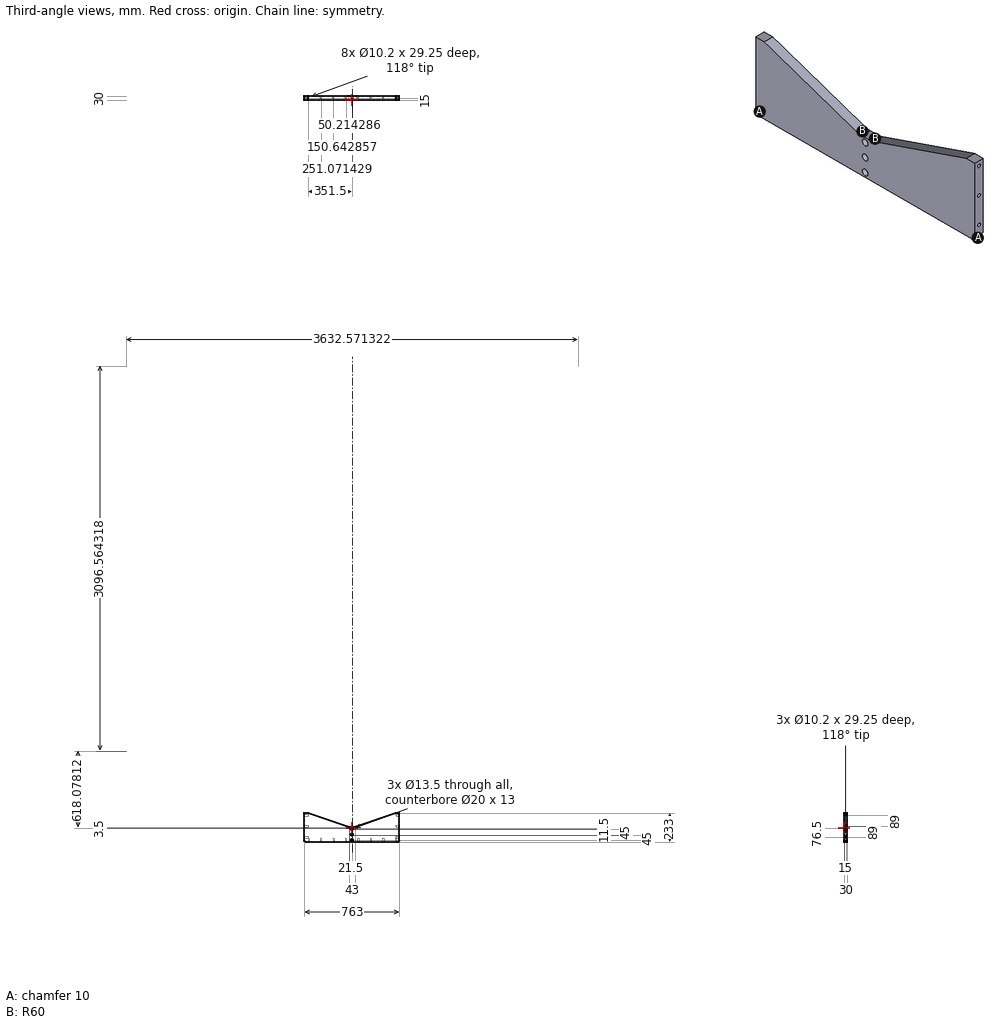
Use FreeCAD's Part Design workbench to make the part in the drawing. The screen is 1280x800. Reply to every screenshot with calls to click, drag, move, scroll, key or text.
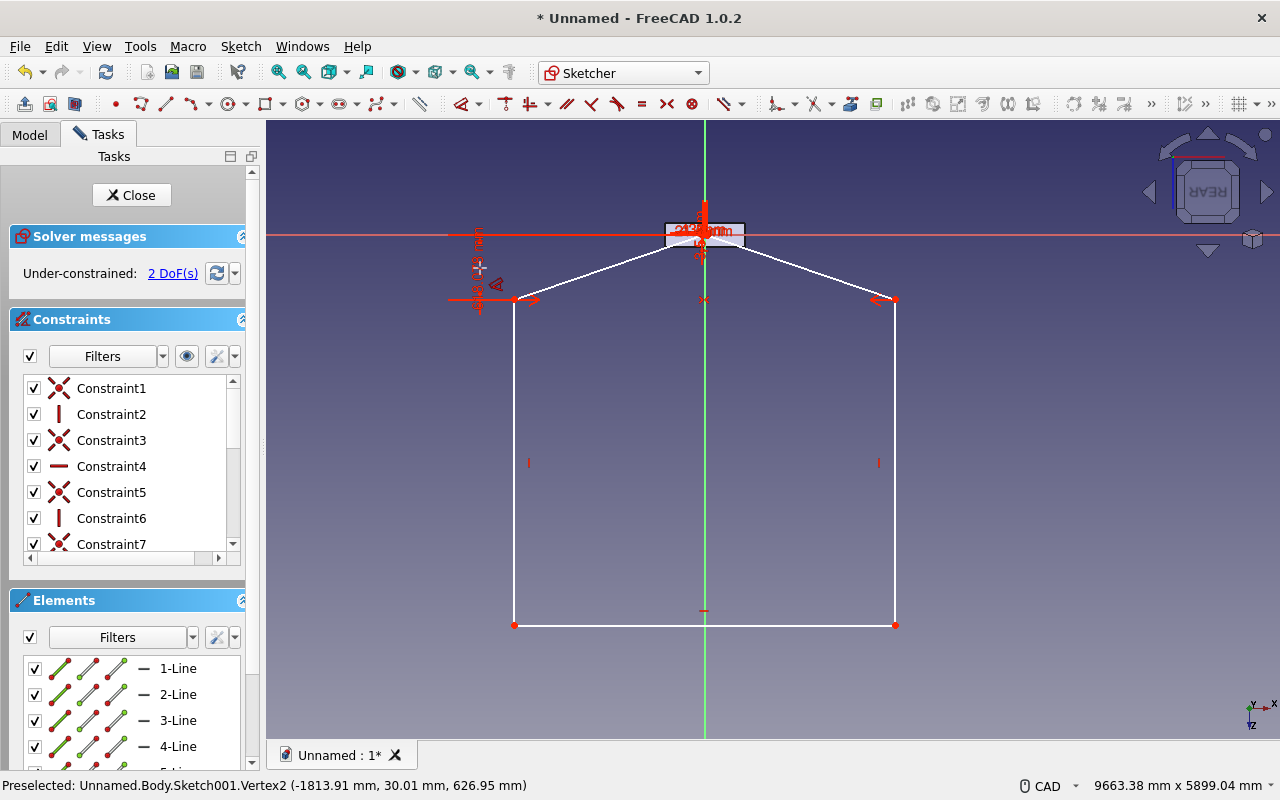
click(514, 398)
click(480, 463)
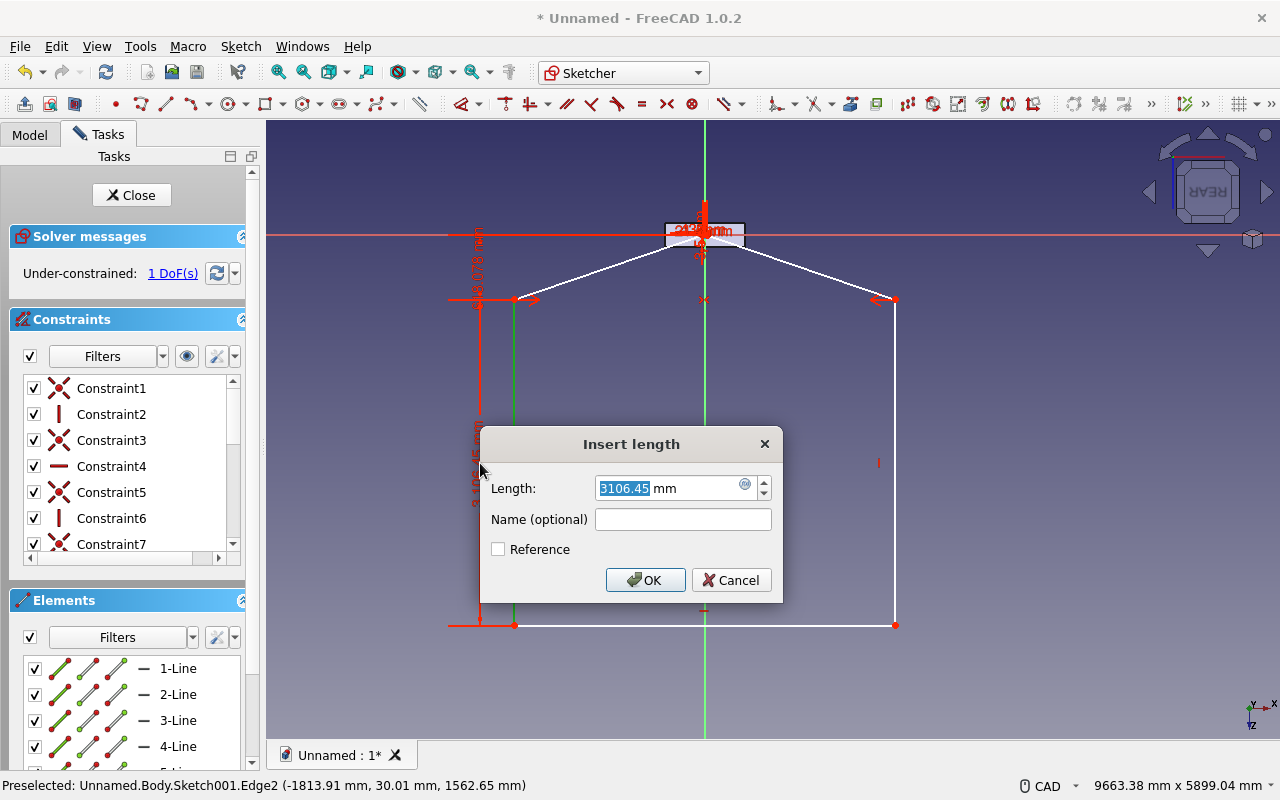
text(3096.564318)
key(Return)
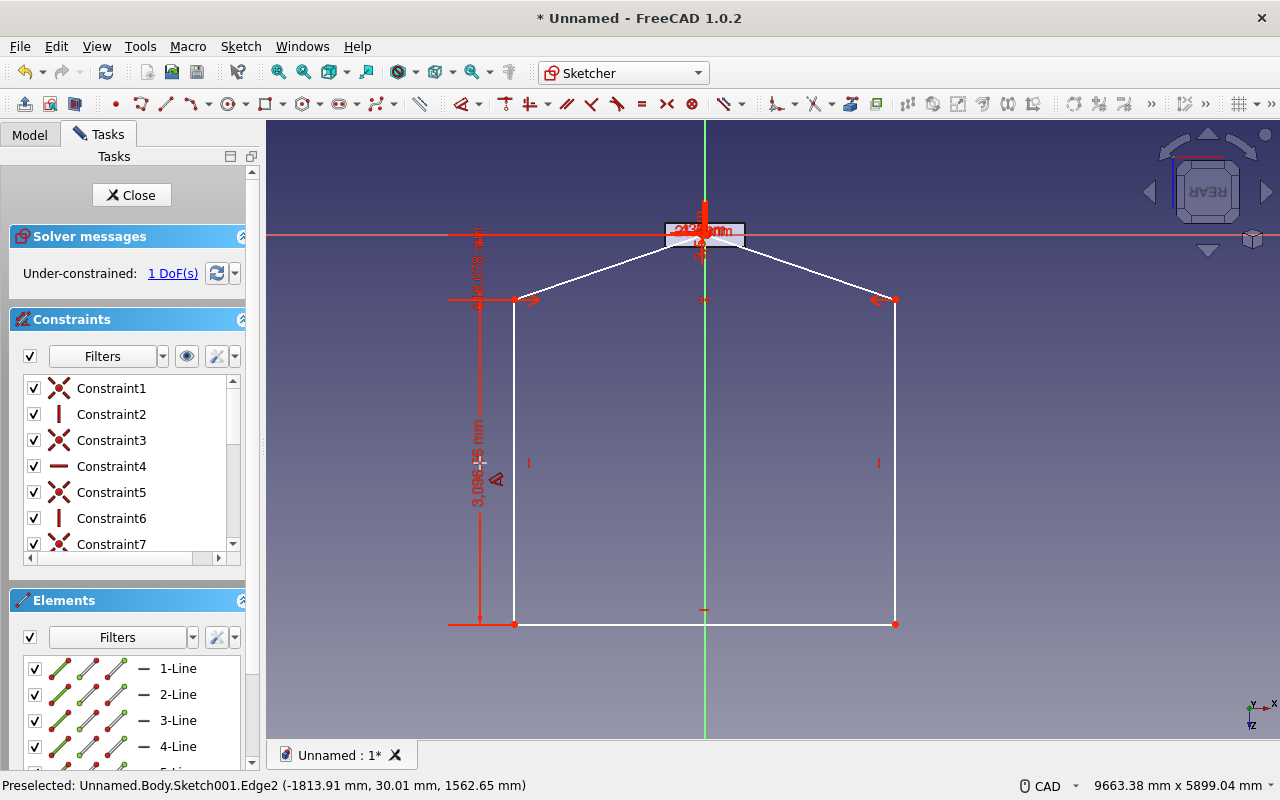
click(629, 625)
click(617, 659)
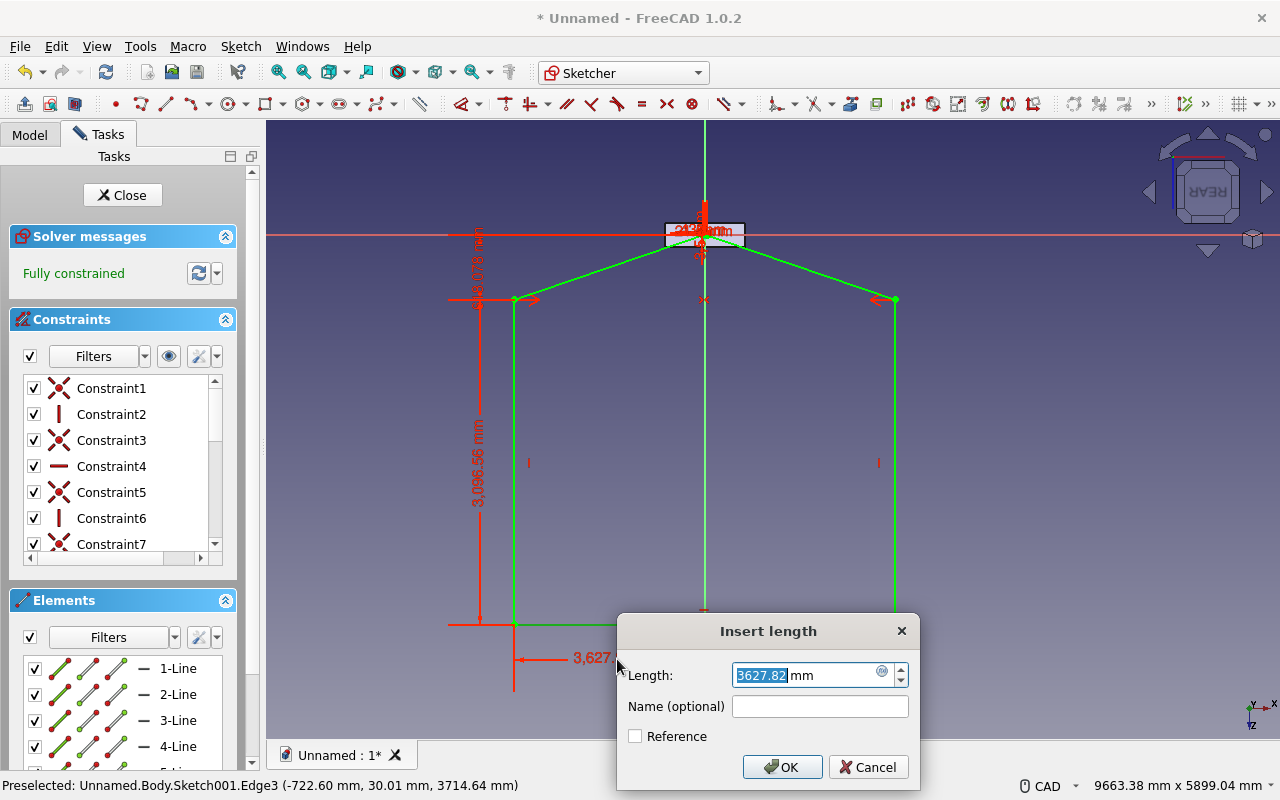
text(3632.571322)
key(Return)
key(Escape)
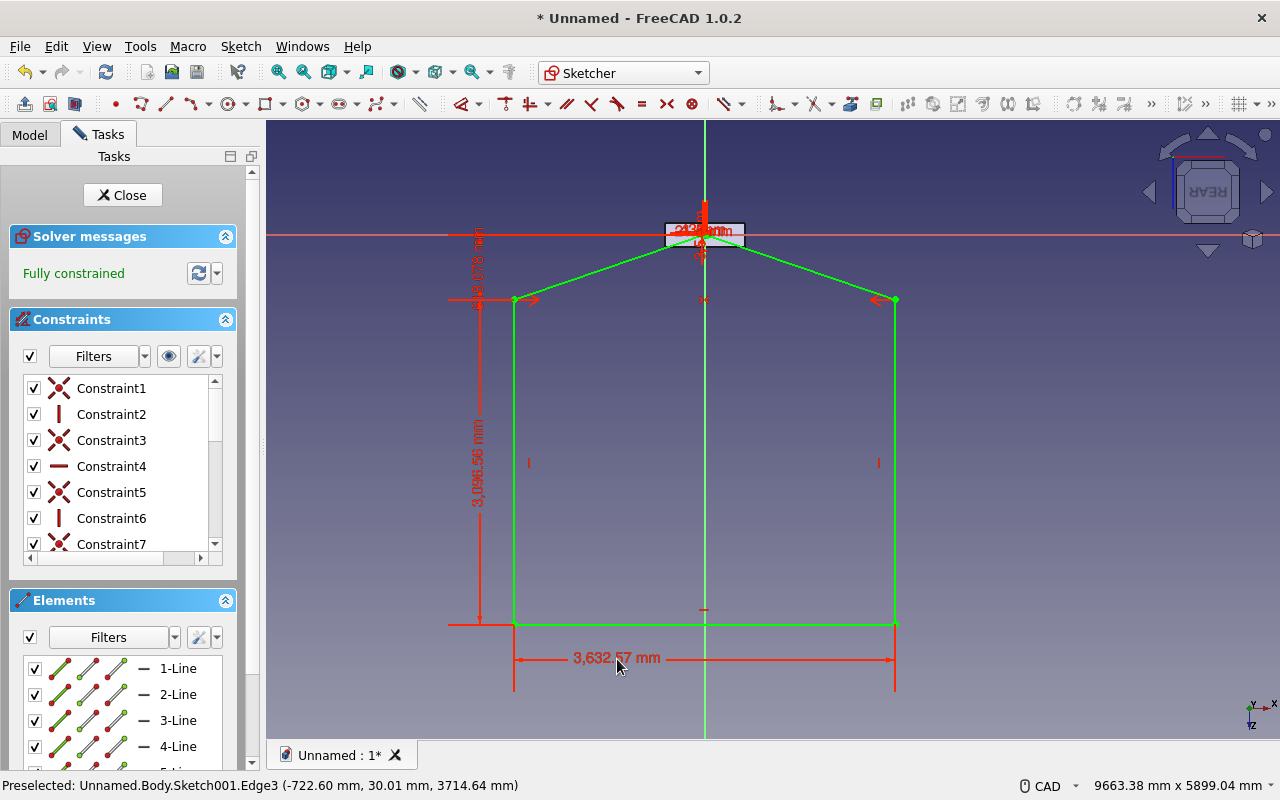
click(123, 195)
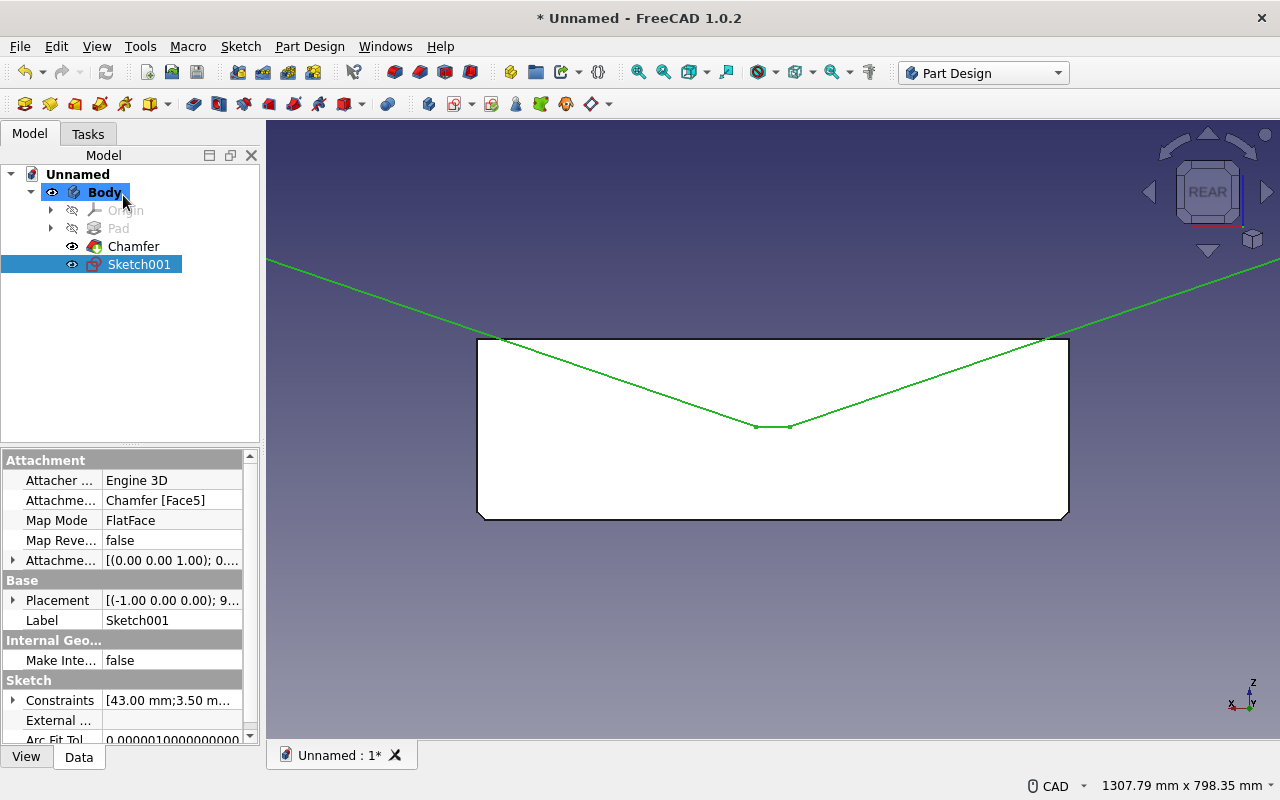
click(194, 104)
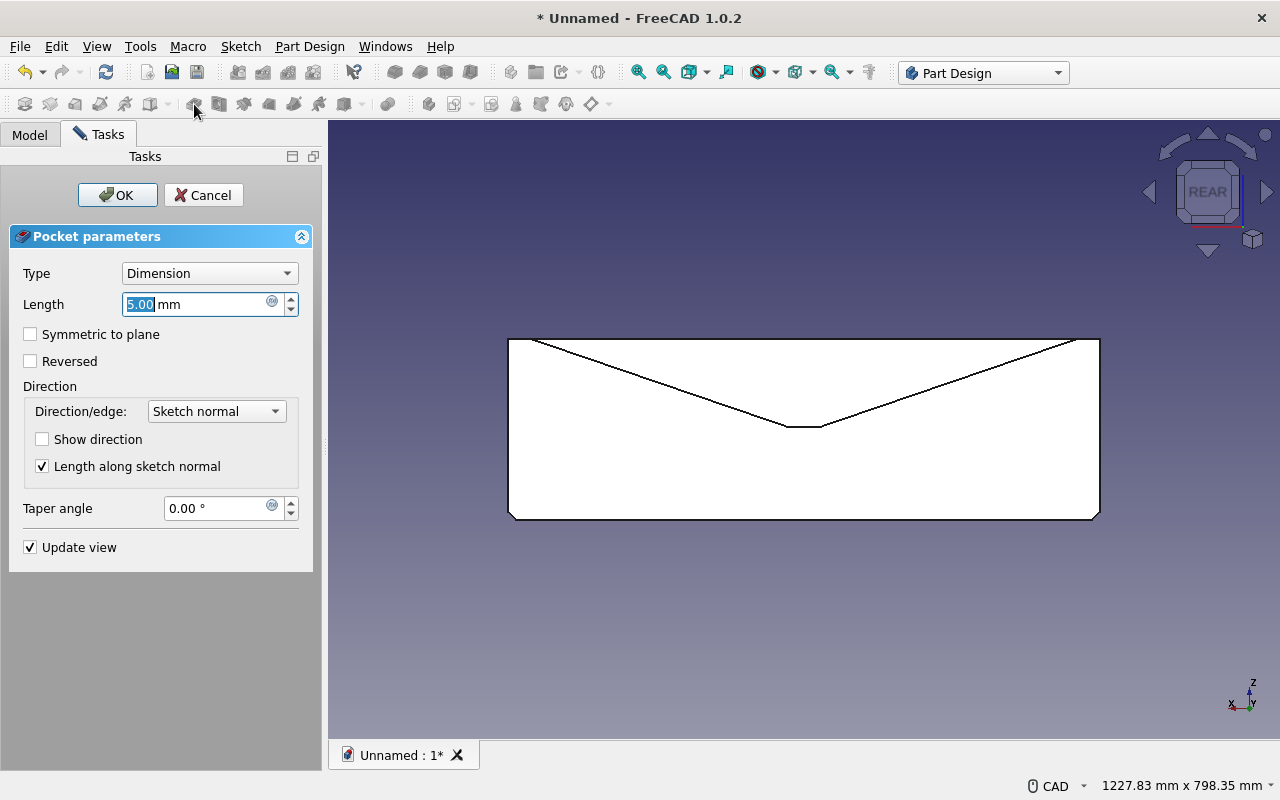
click(210, 274)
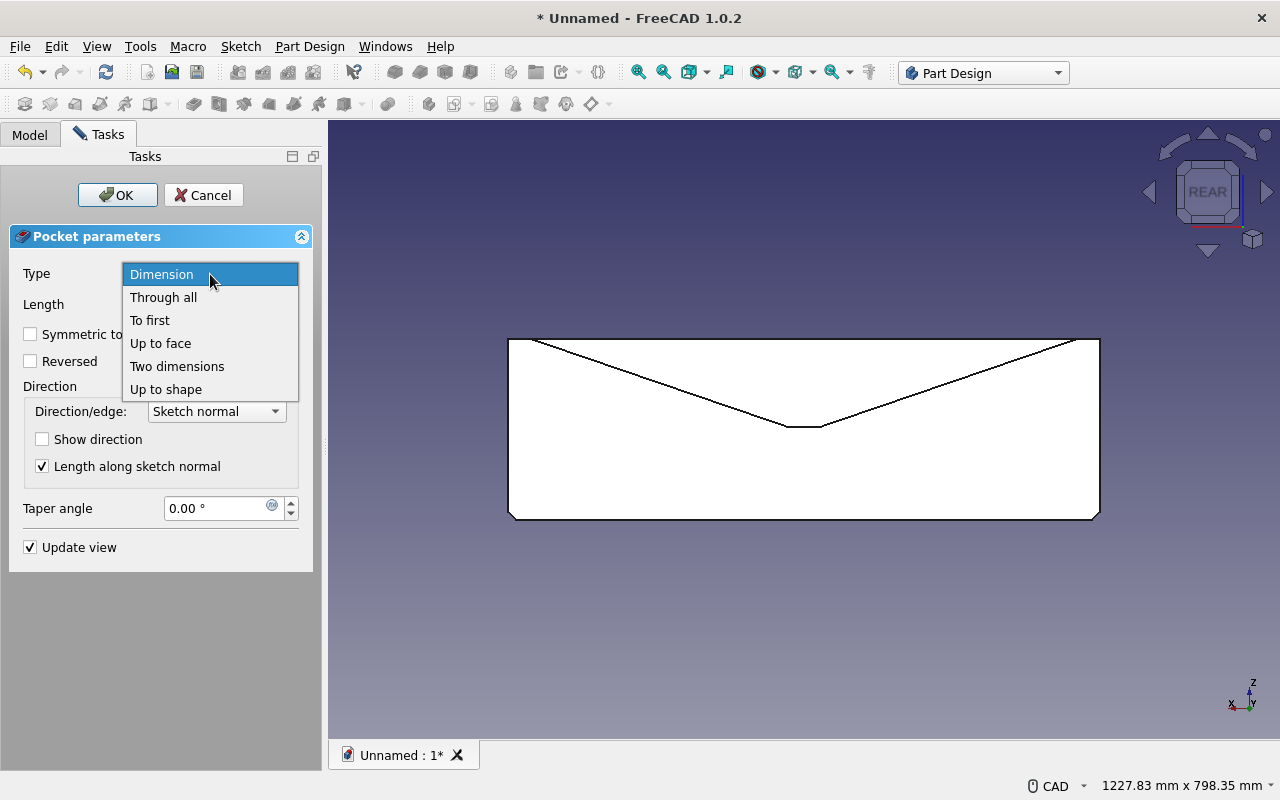
click(208, 366)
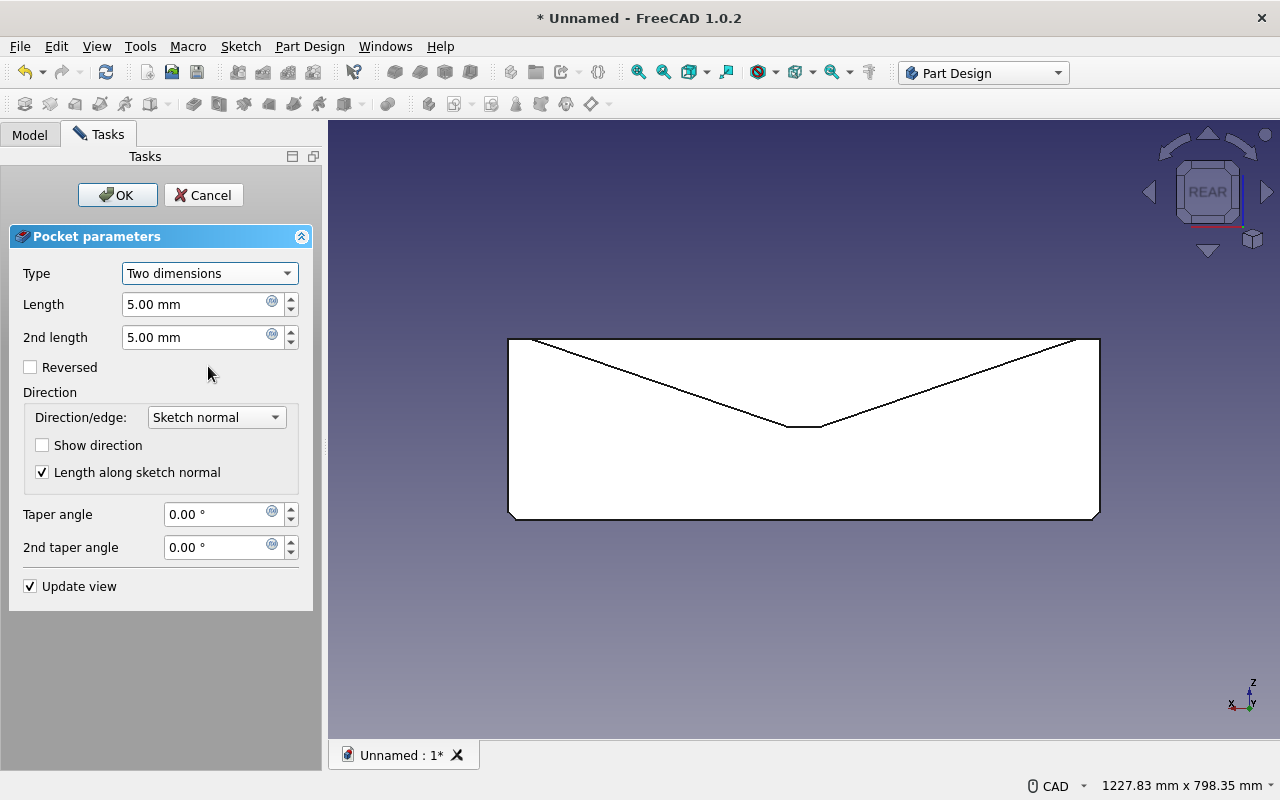
triple_click(204, 304)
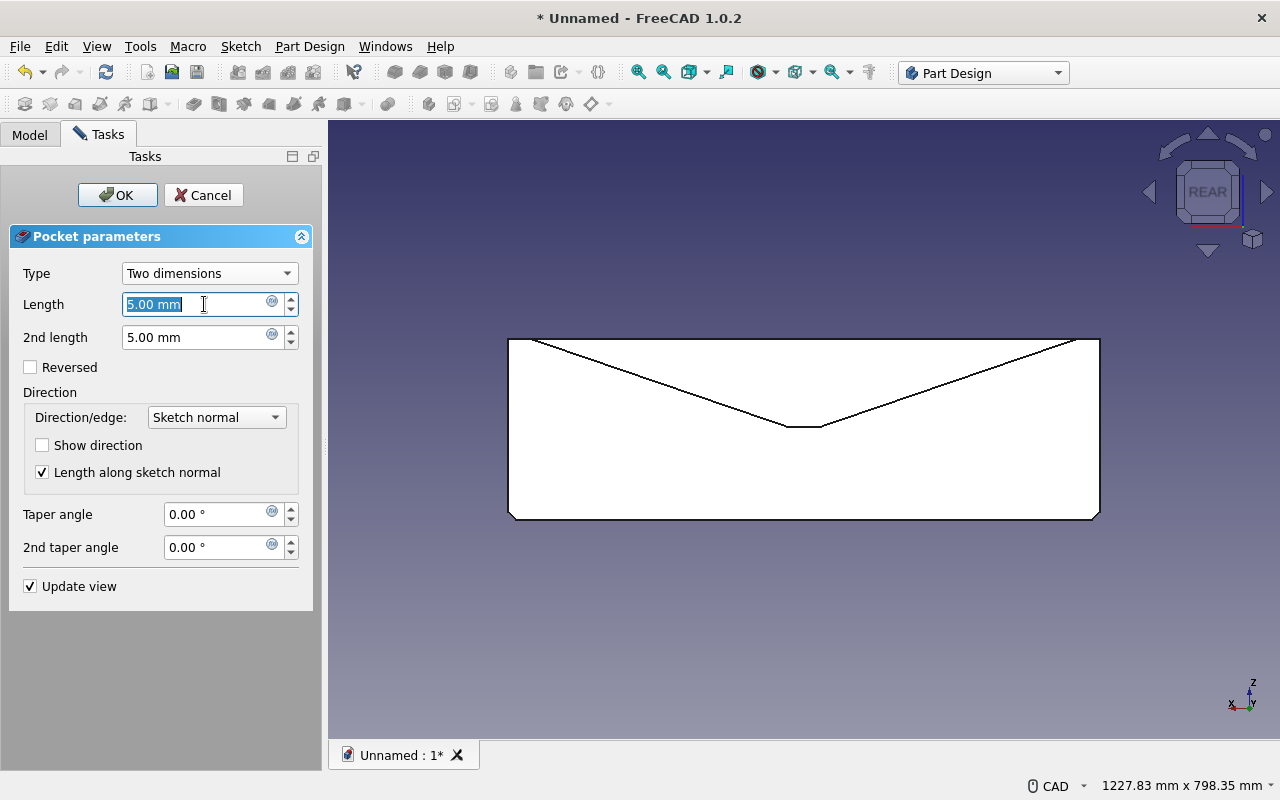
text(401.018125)
key(Tab)